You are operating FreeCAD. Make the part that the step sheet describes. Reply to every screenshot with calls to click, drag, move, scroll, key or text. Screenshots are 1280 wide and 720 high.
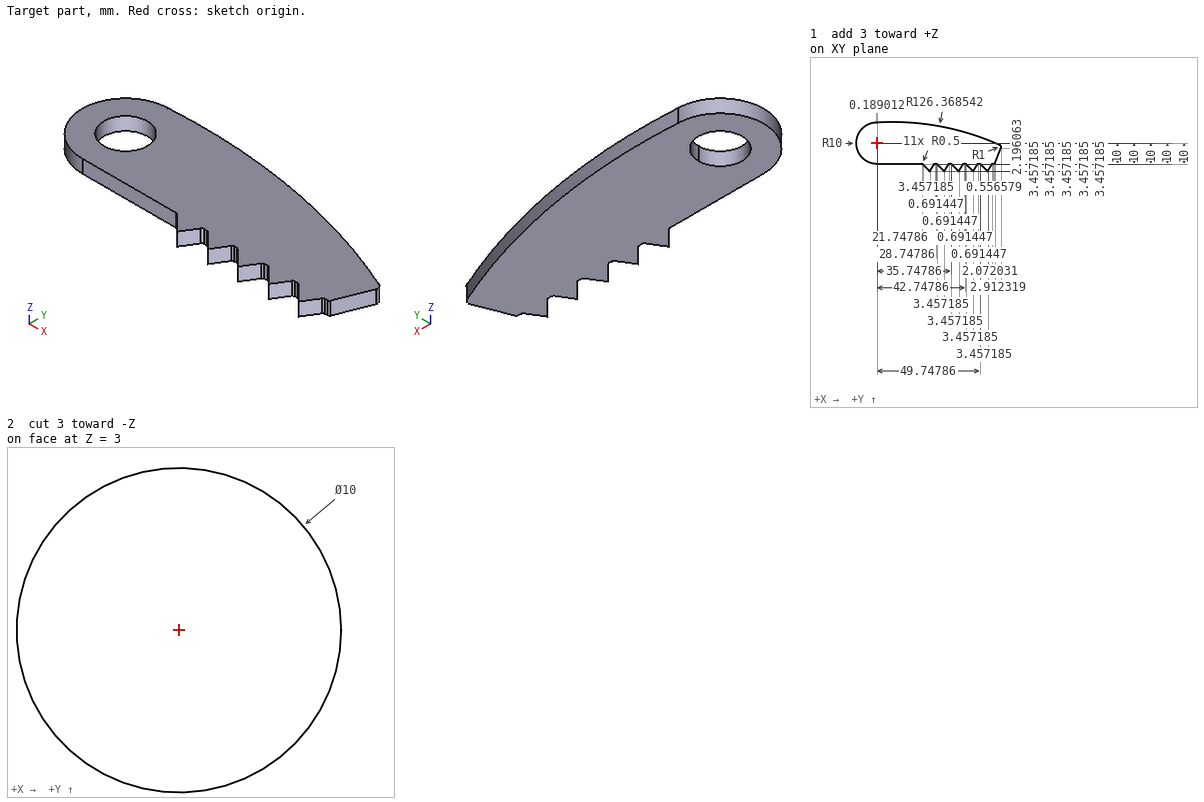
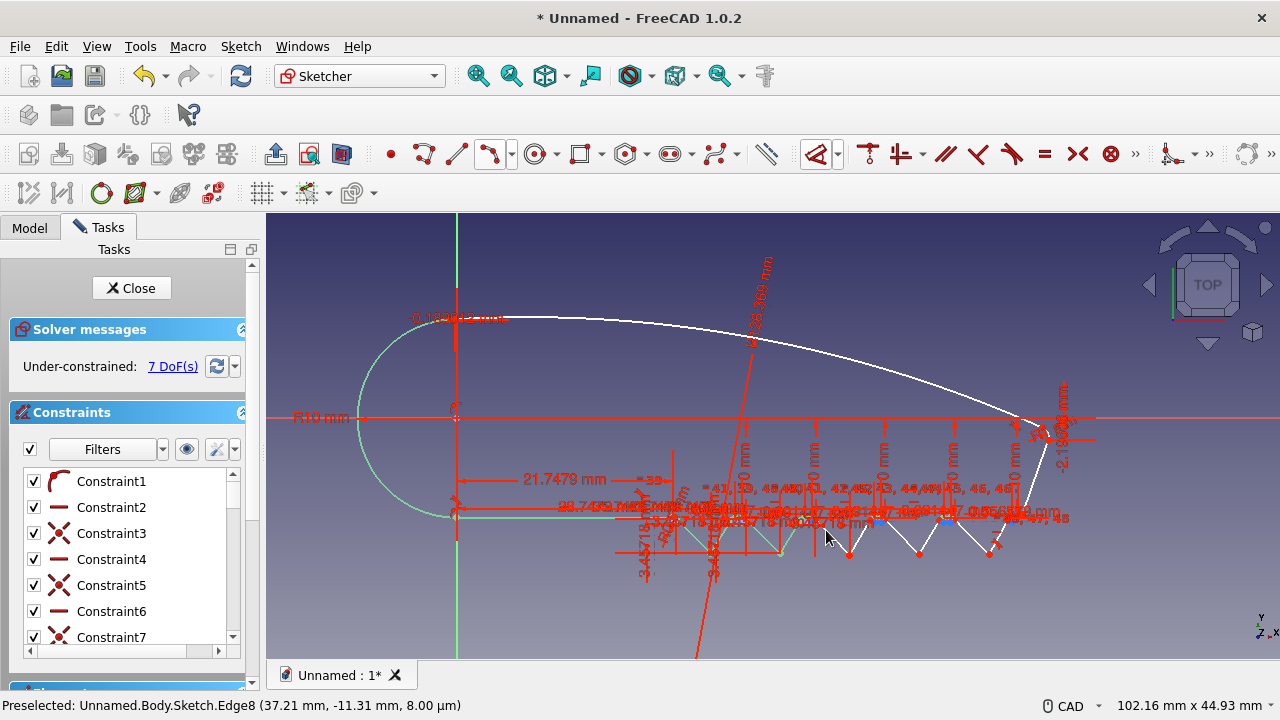
click(839, 544)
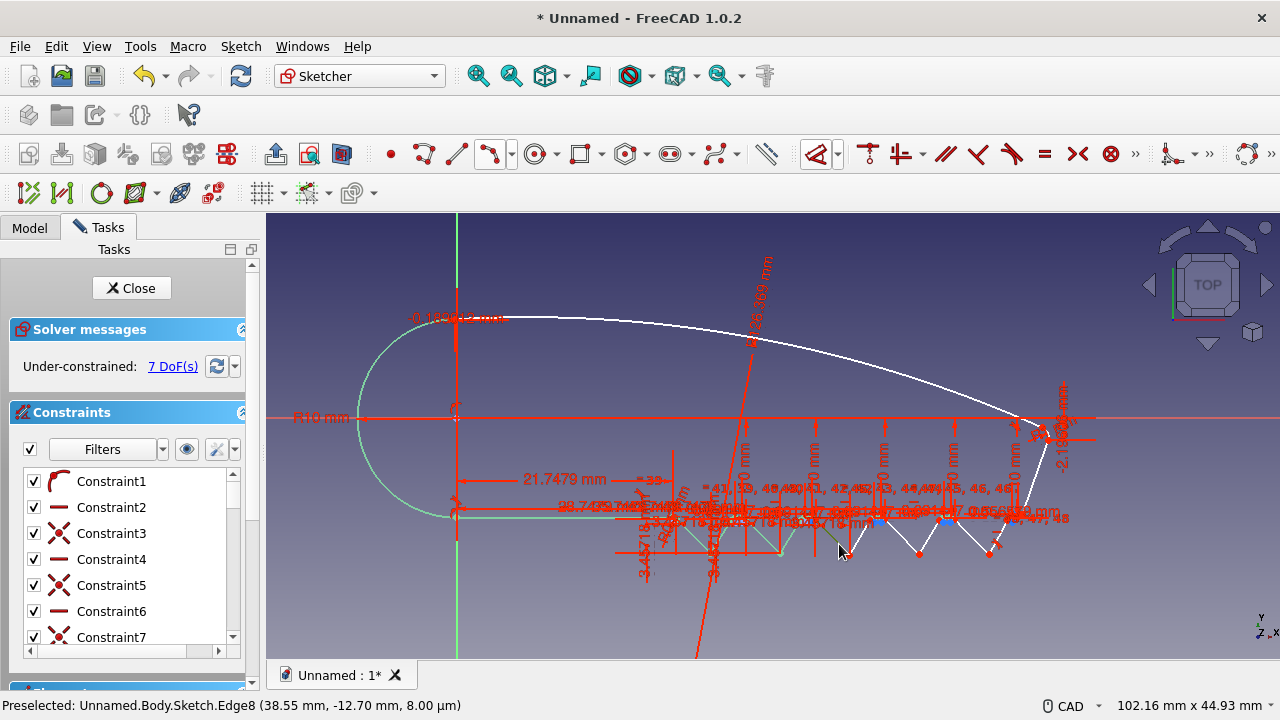
key(i)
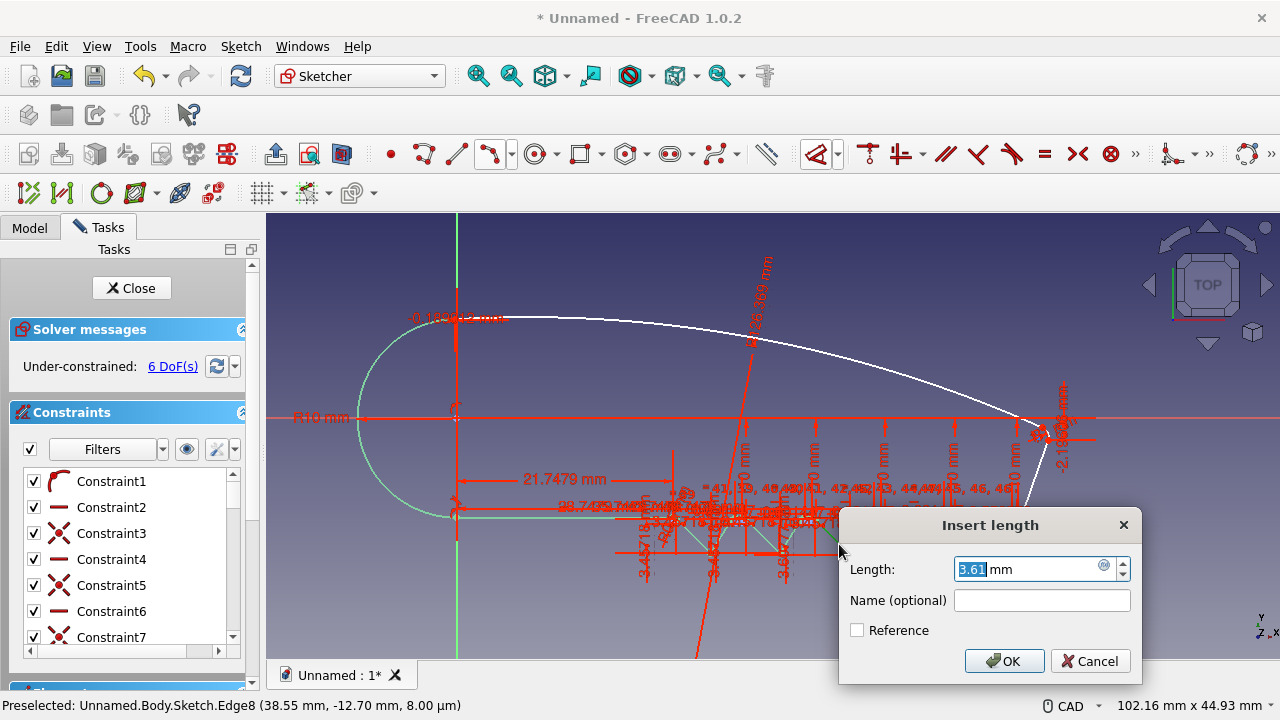
text(3.457185)
key(Return)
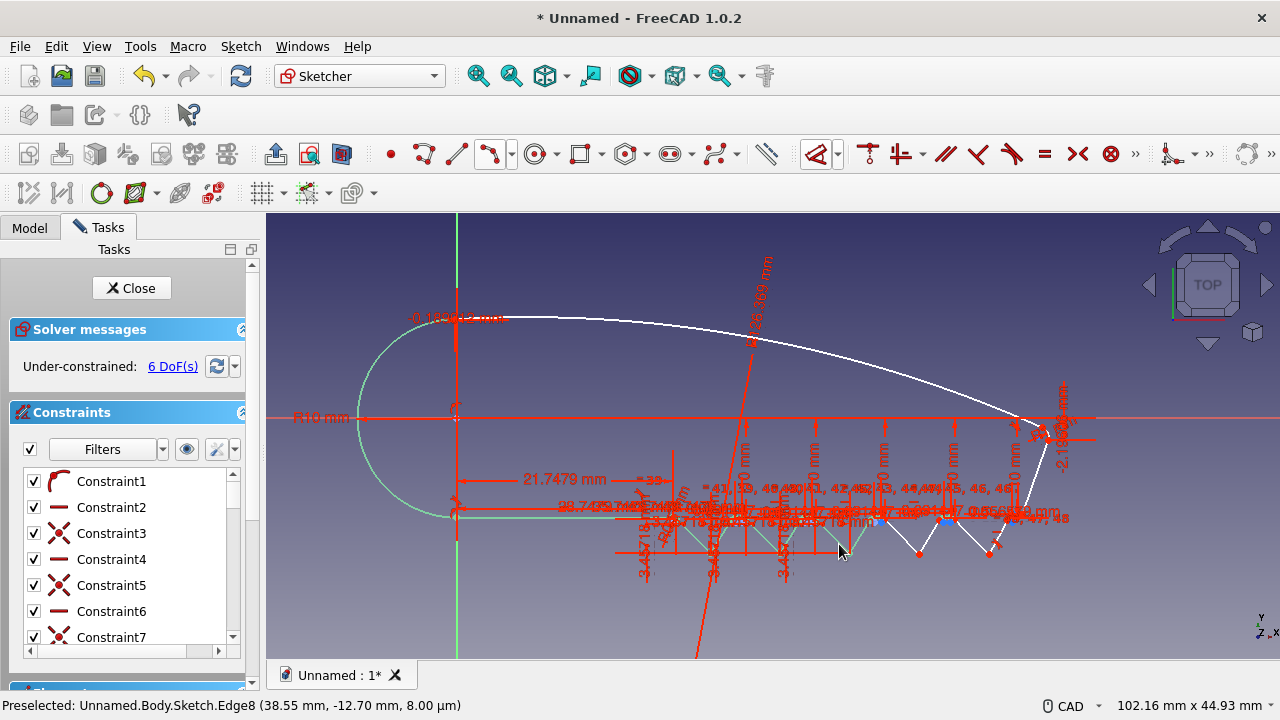
click(895, 530)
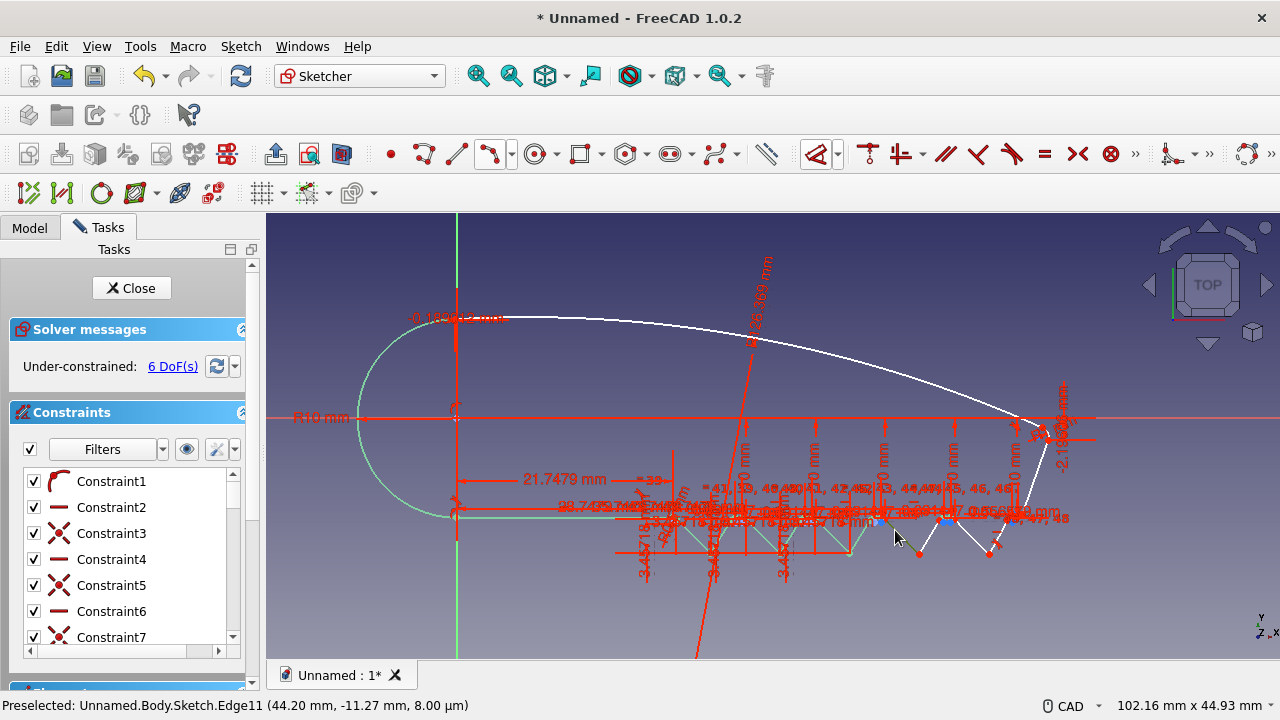
key(l)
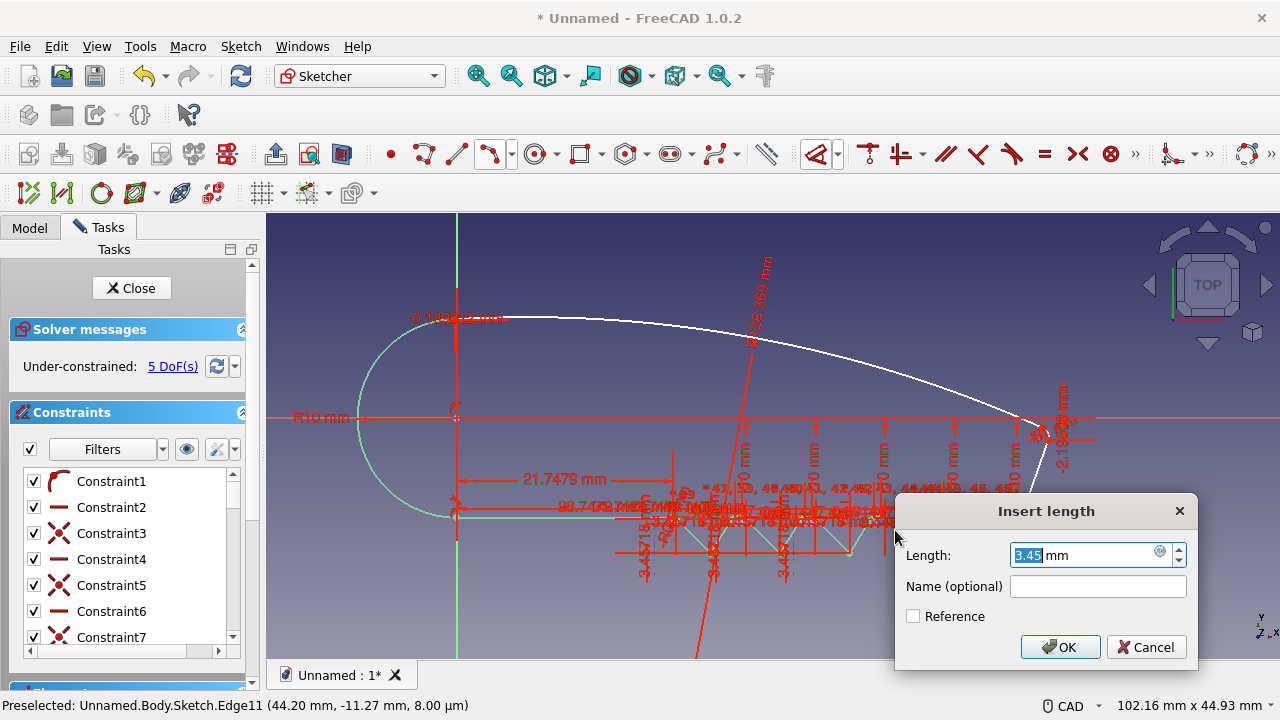
text(3.457185)
key(Return)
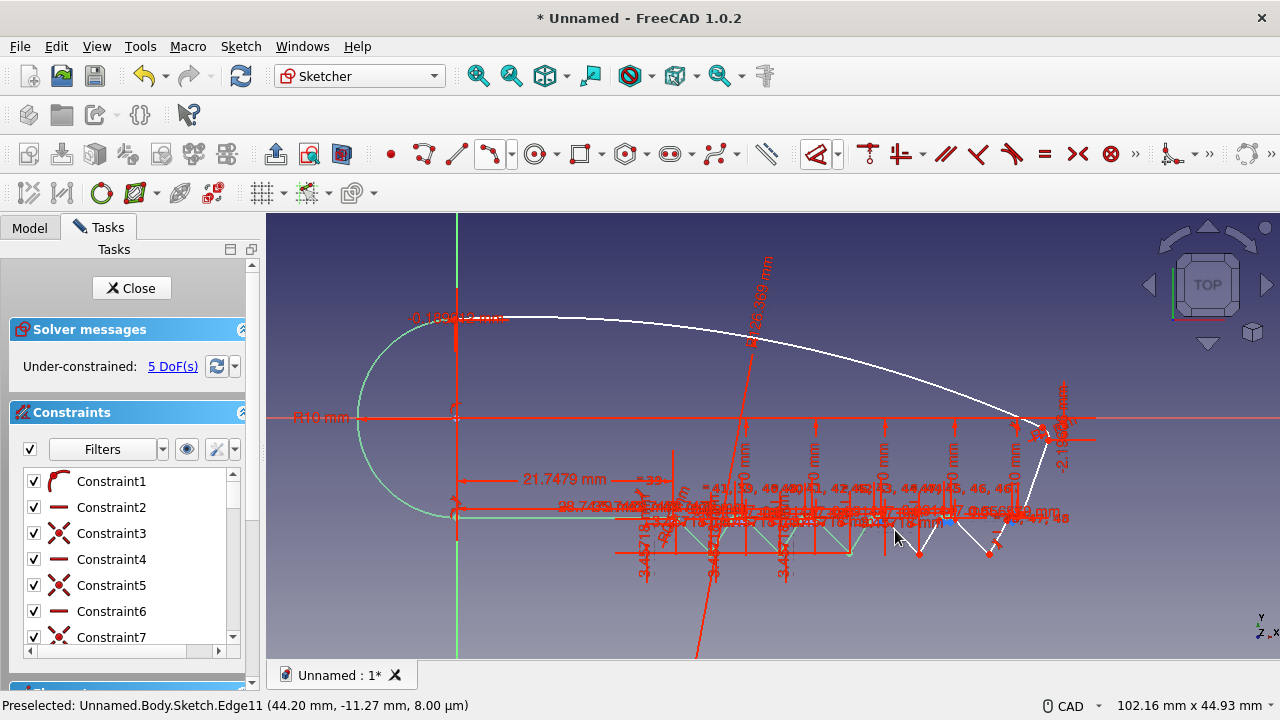
click(909, 544)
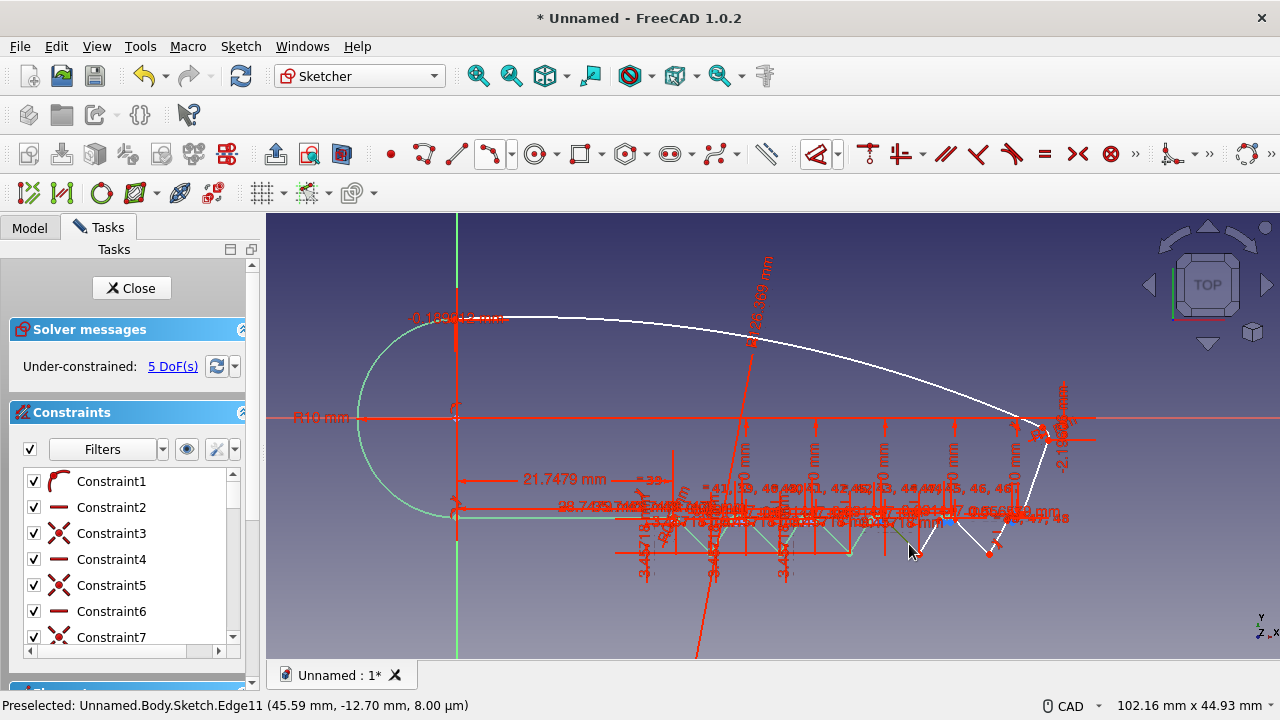
key(i)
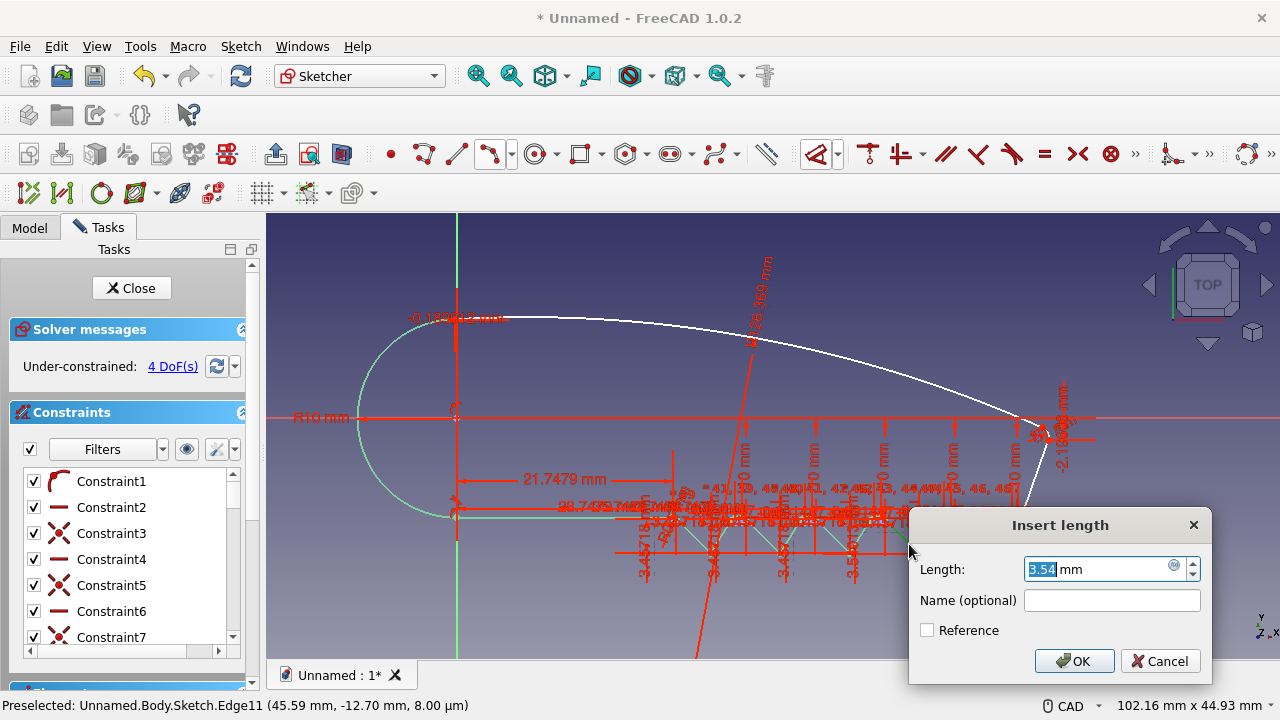
text(3.457185)
key(Return)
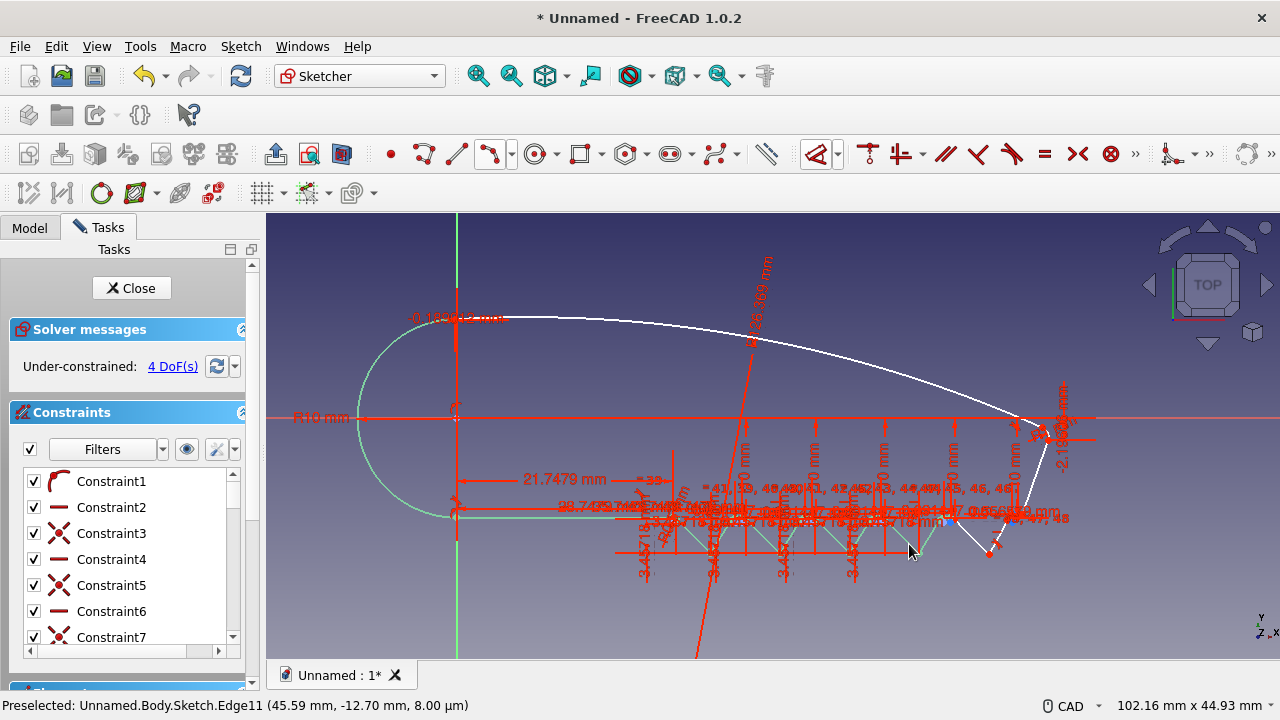
click(965, 530)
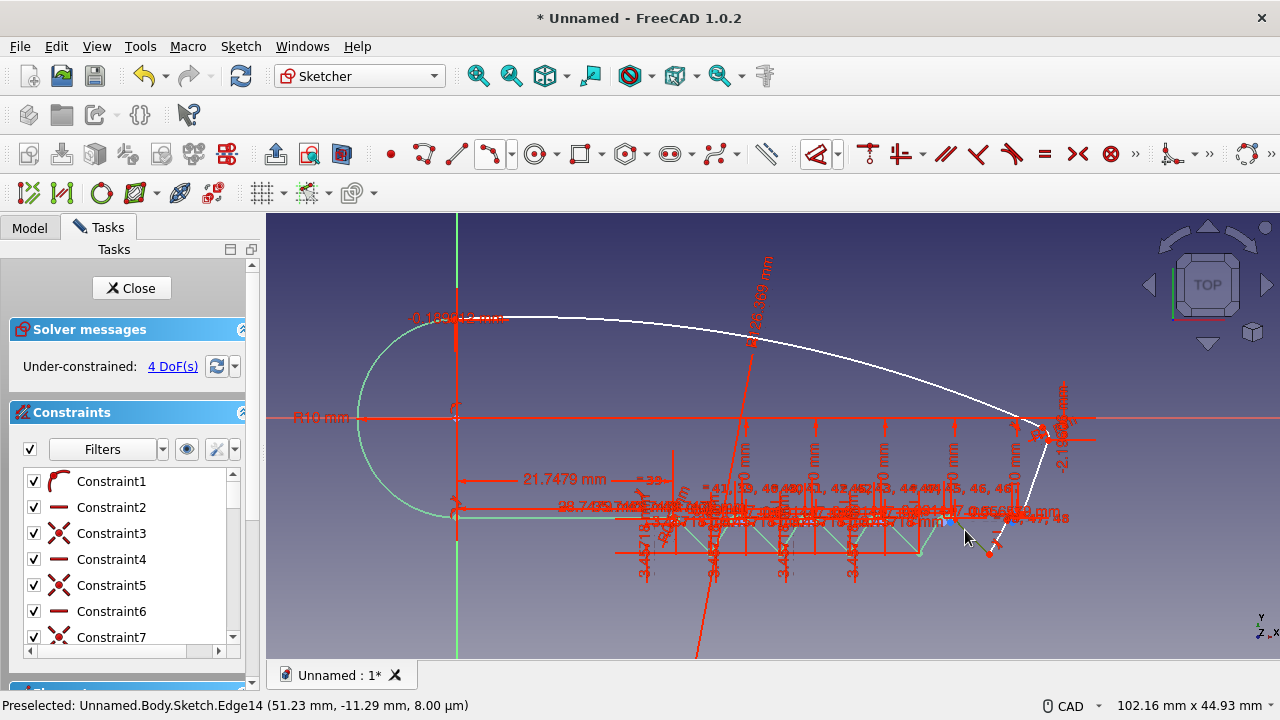
key(l)